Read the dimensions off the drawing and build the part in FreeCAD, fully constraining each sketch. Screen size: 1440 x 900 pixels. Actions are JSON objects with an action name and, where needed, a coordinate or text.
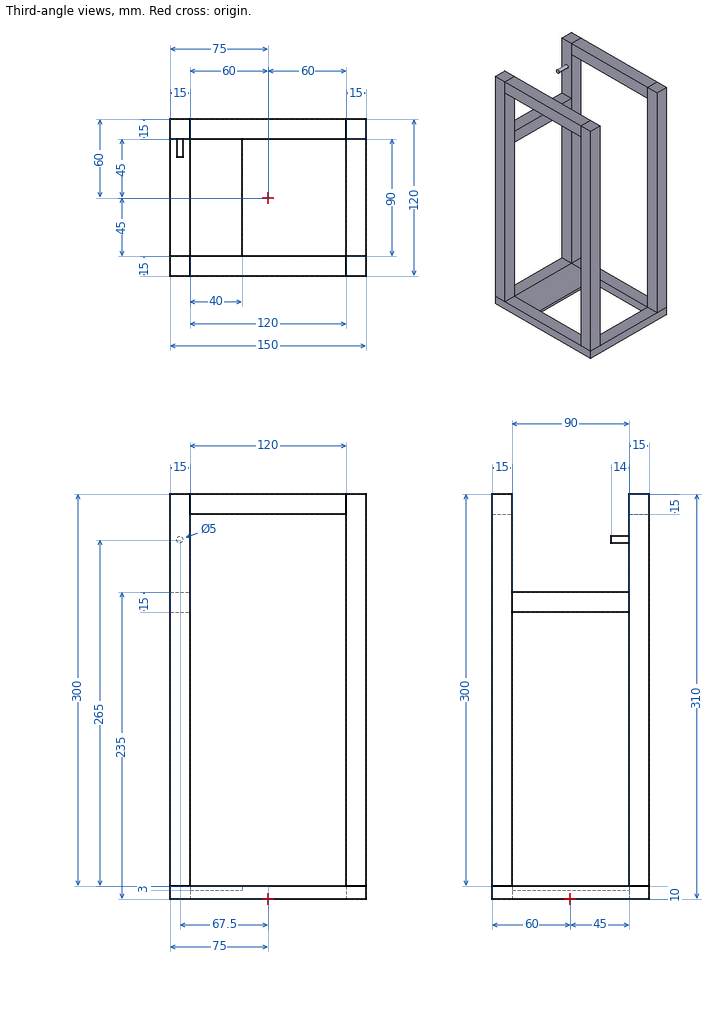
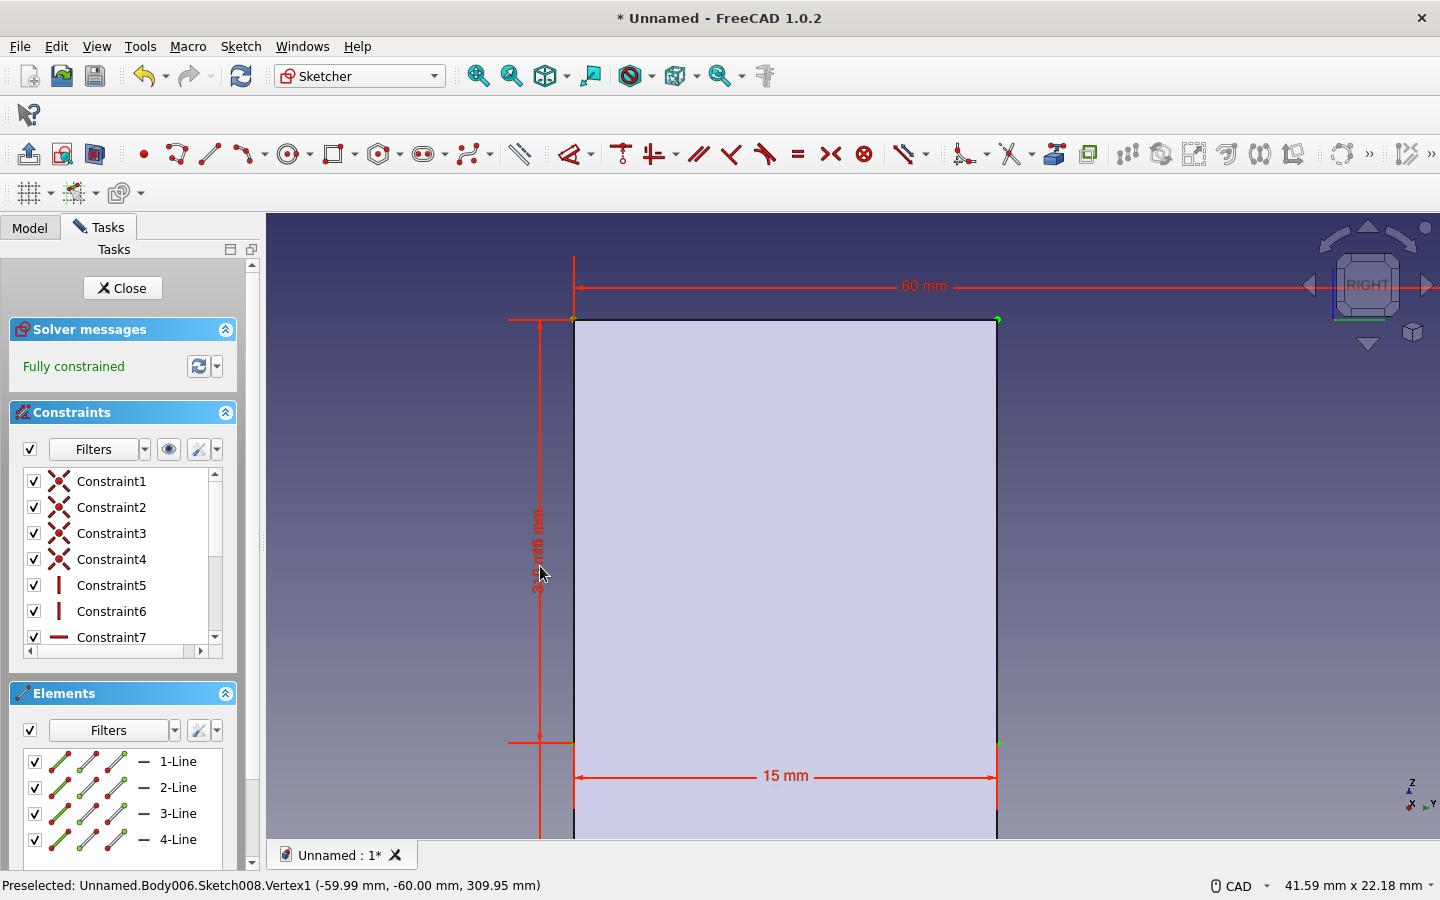
{"action": "left_click", "coordinate": [123, 288]}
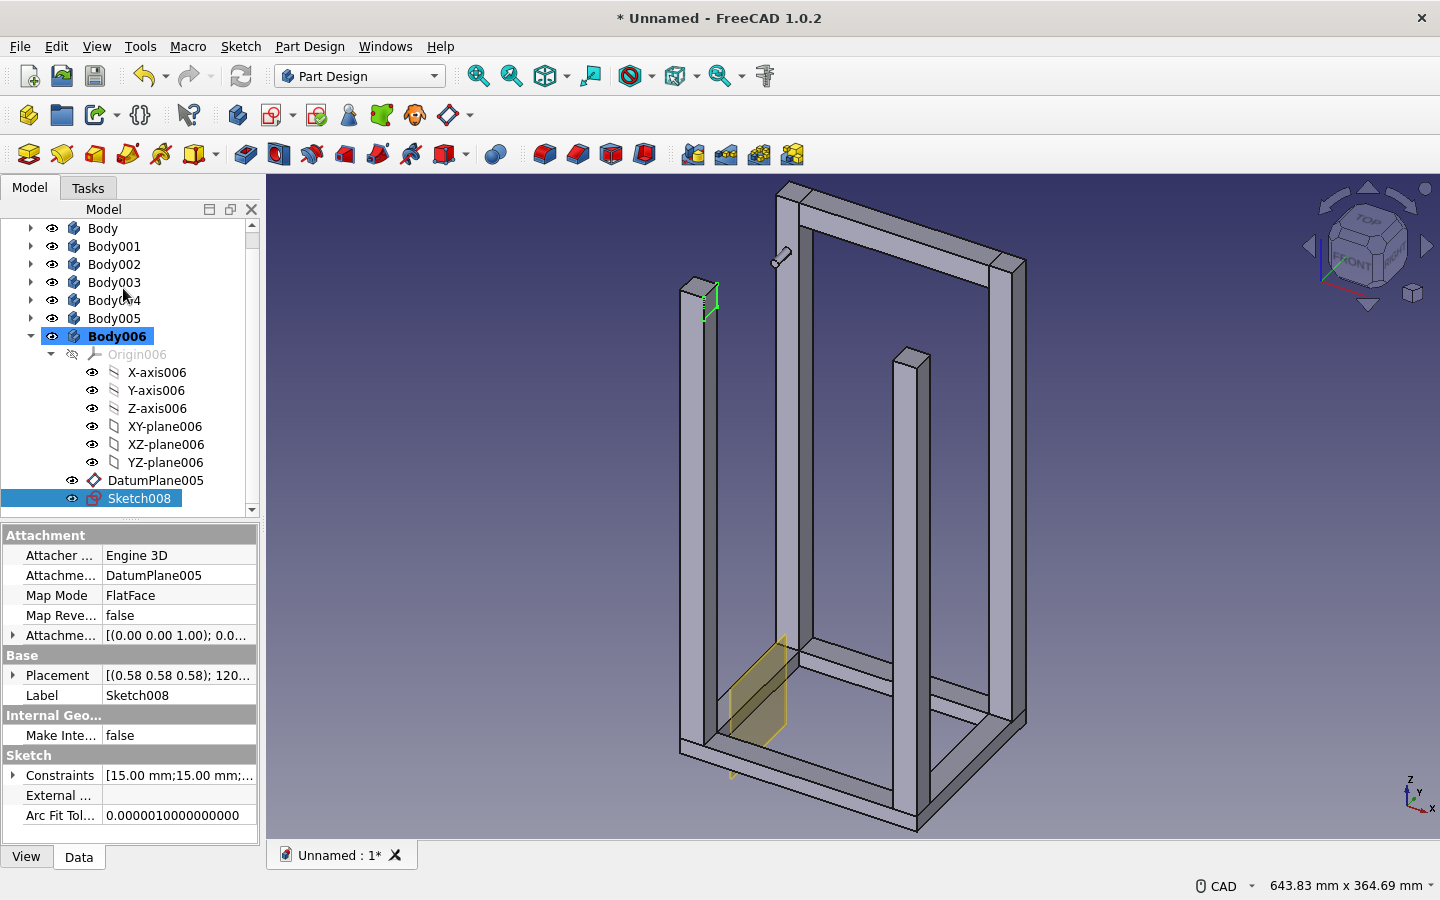
{"action": "left_click", "coordinate": [29, 154]}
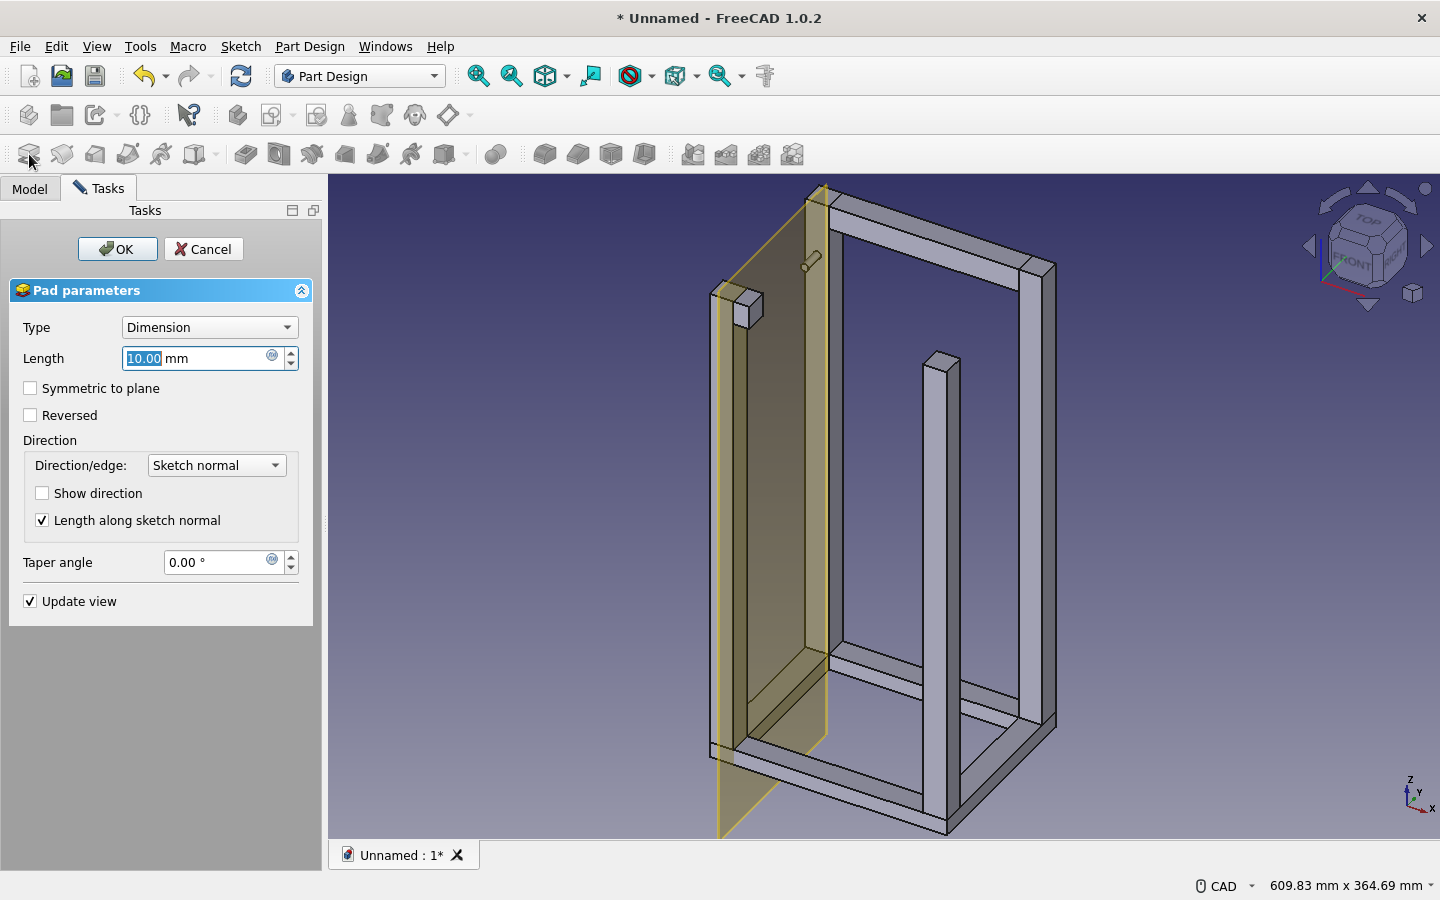
{"action": "type", "text": "120"}
{"action": "key", "text": "Tab"}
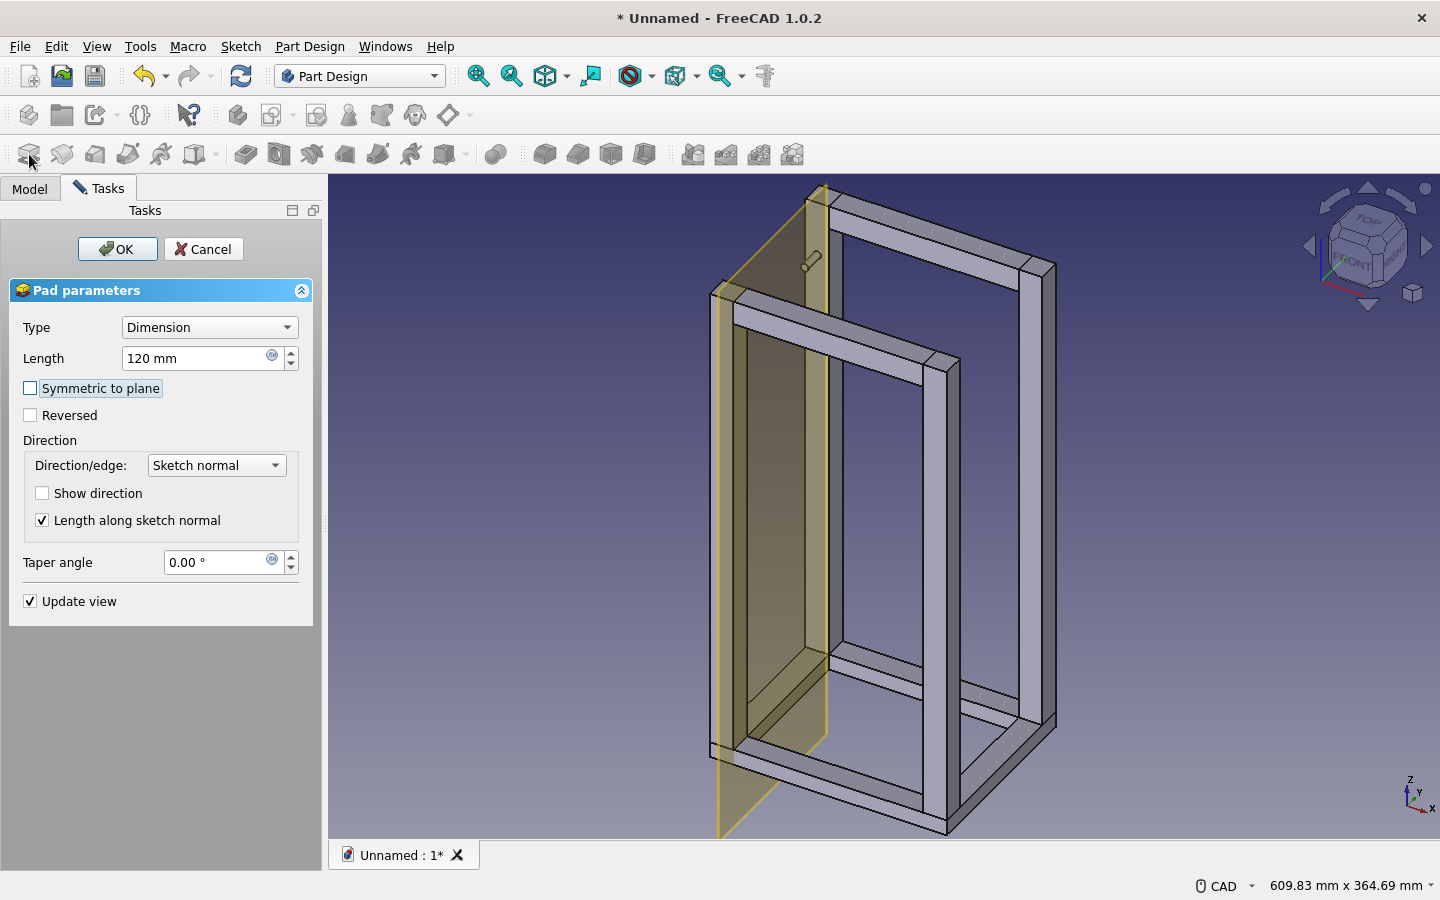
{"action": "left_click", "coordinate": [118, 249]}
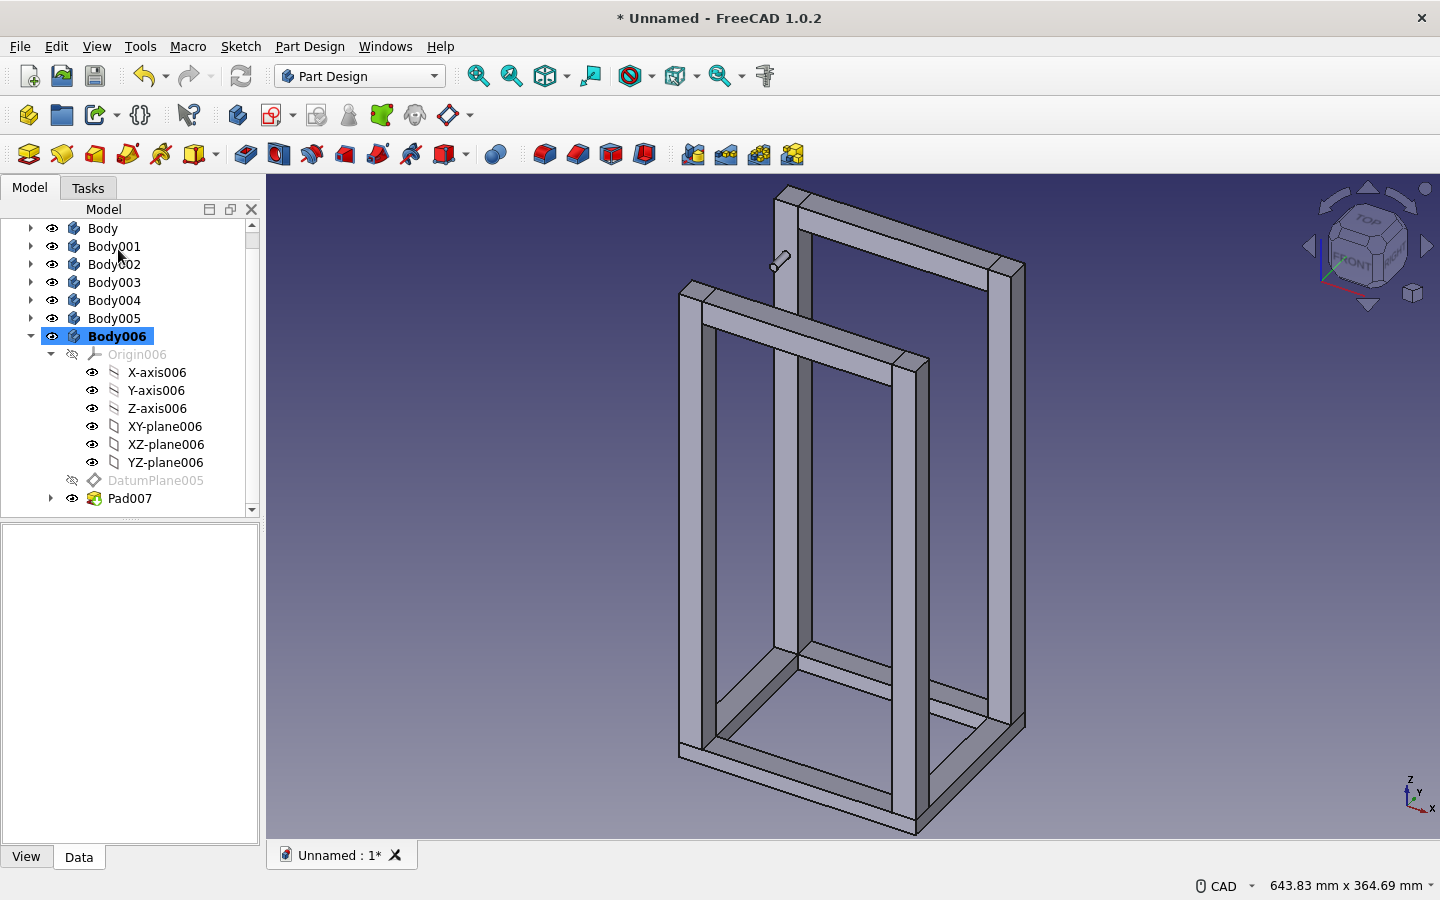
{"action": "left_click", "coordinate": [479, 76]}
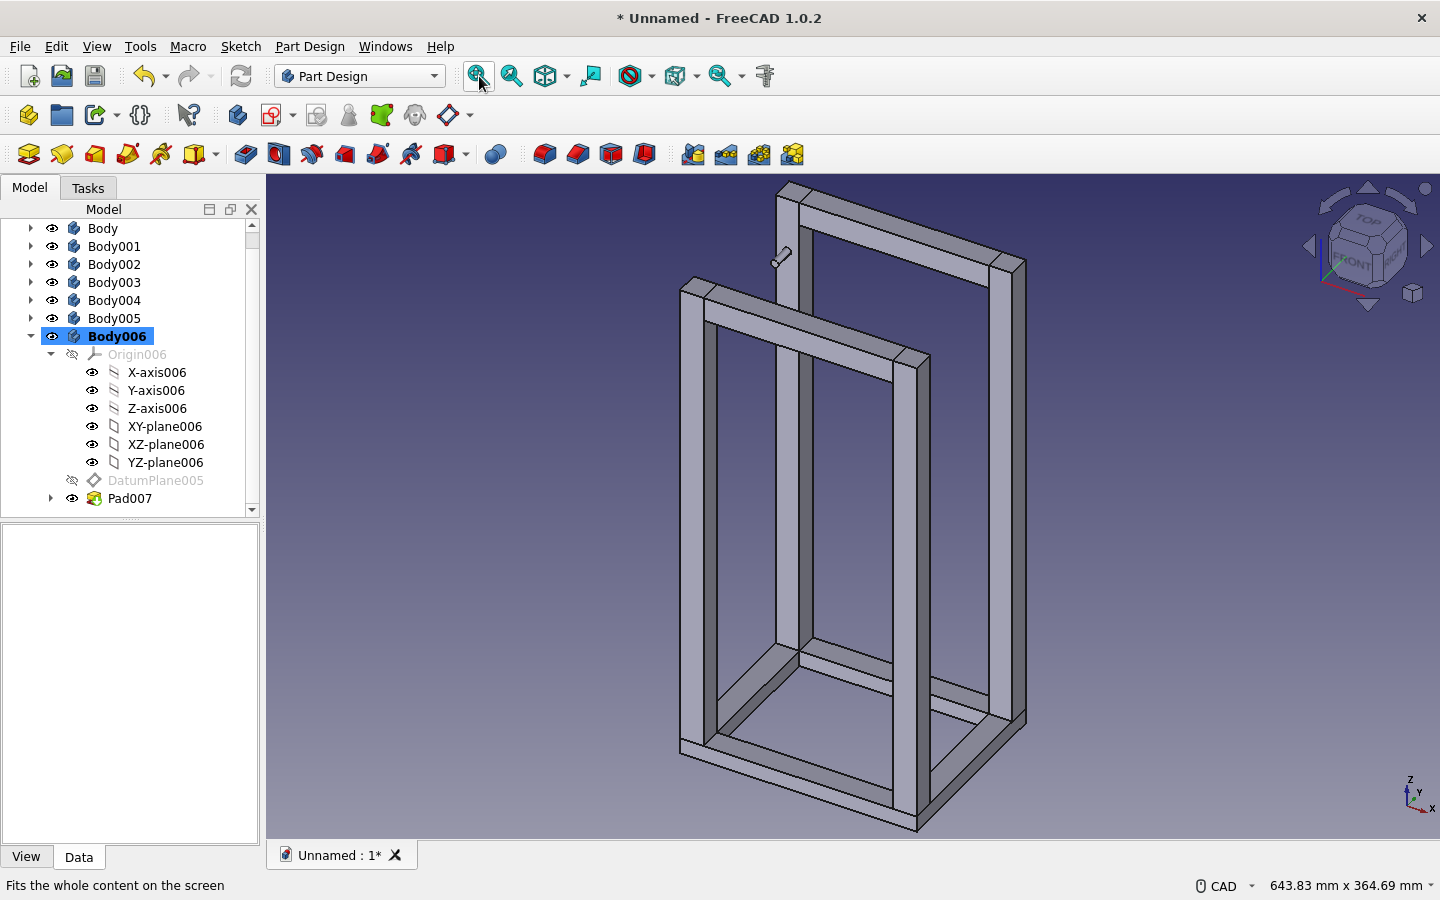
{"action": "left_click", "coordinate": [238, 116]}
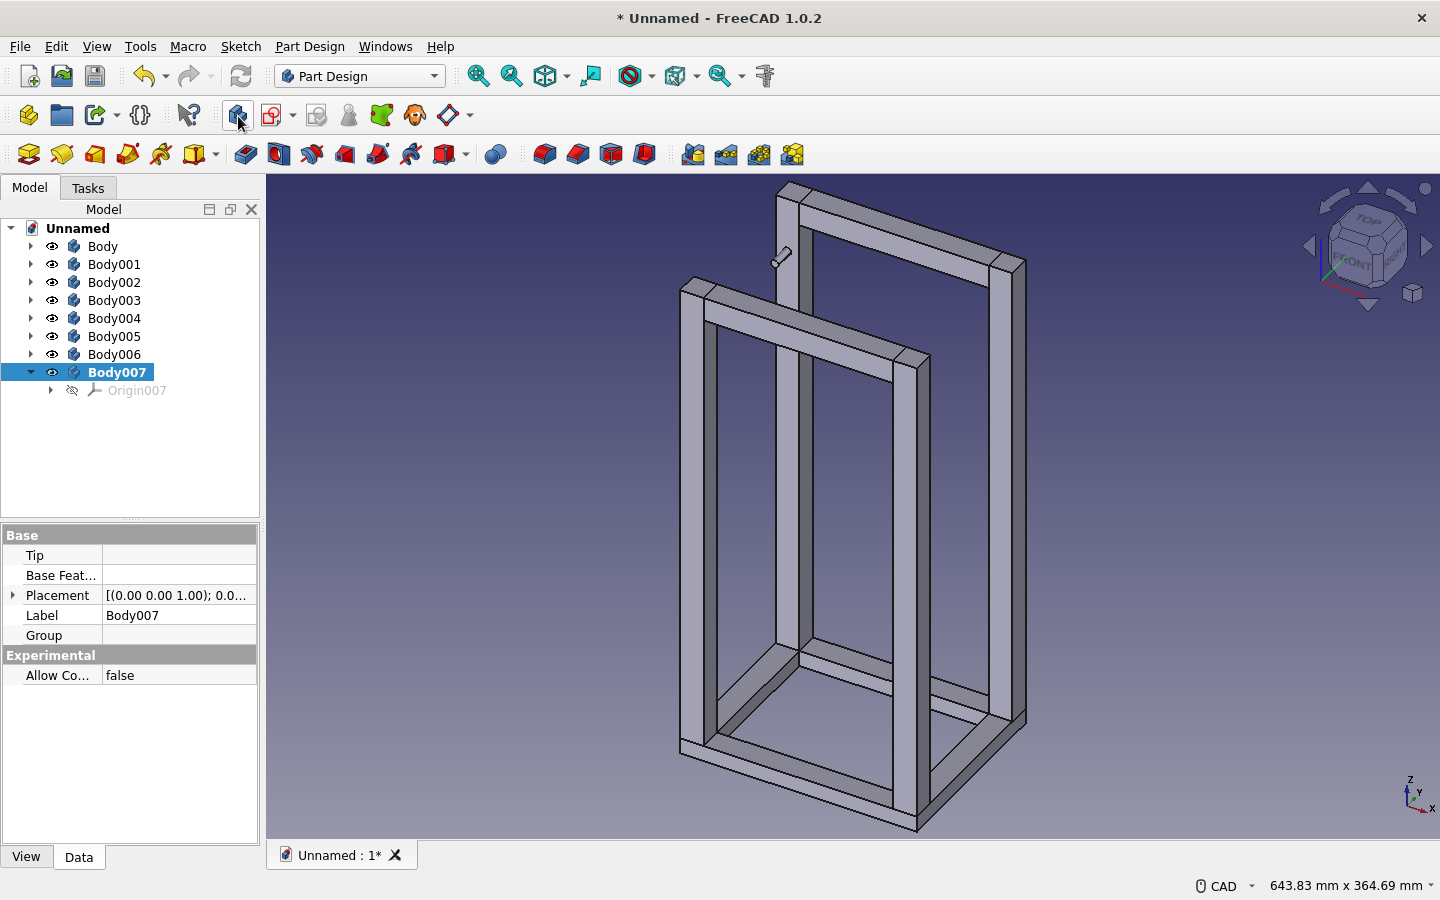
{"action": "left_click", "coordinate": [51, 390]}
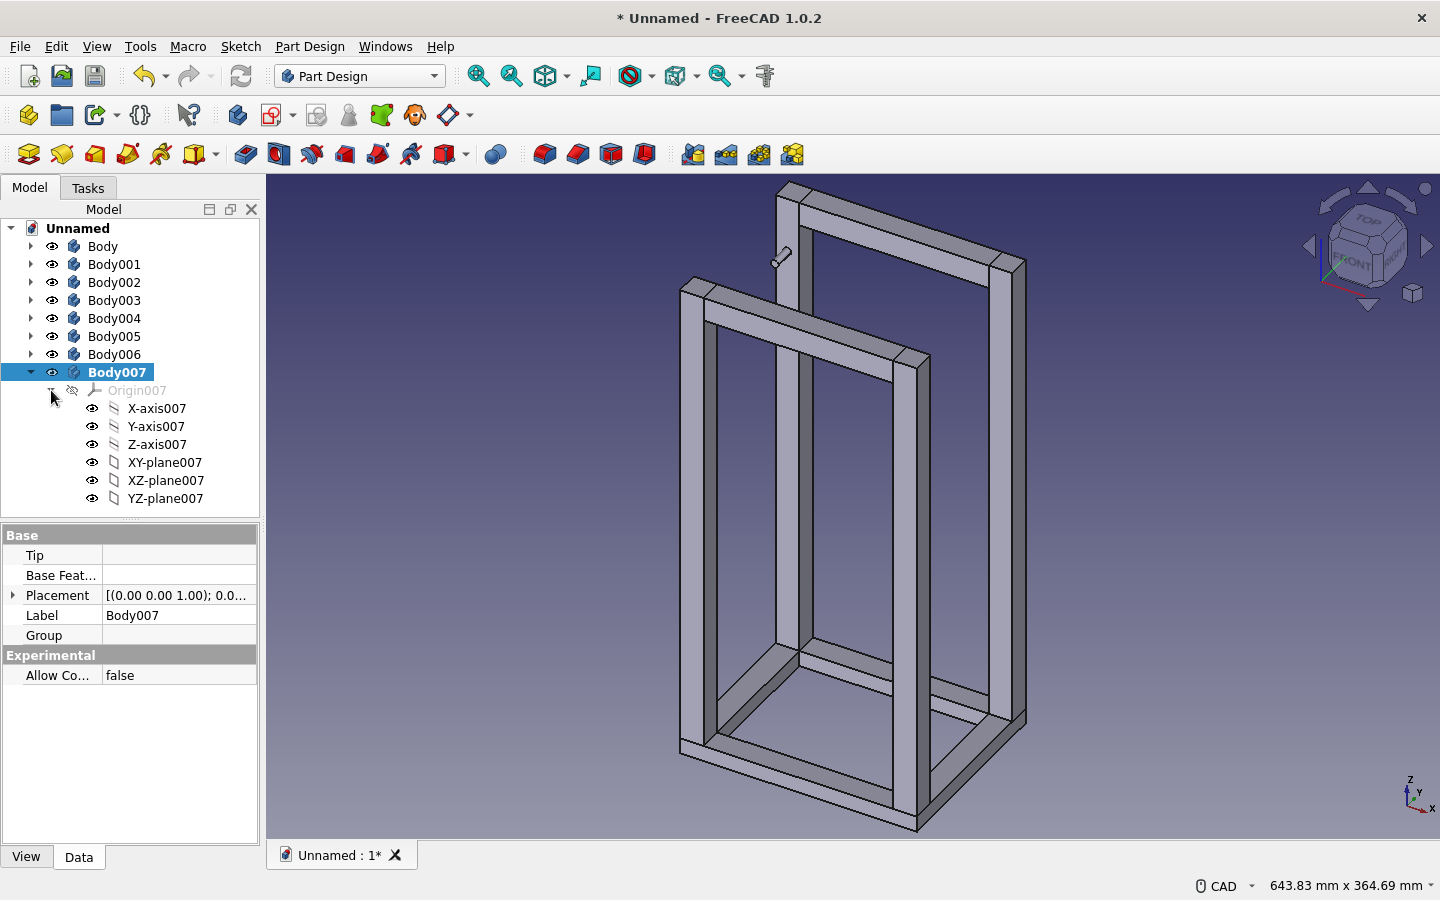
{"action": "left_click", "coordinate": [137, 480]}